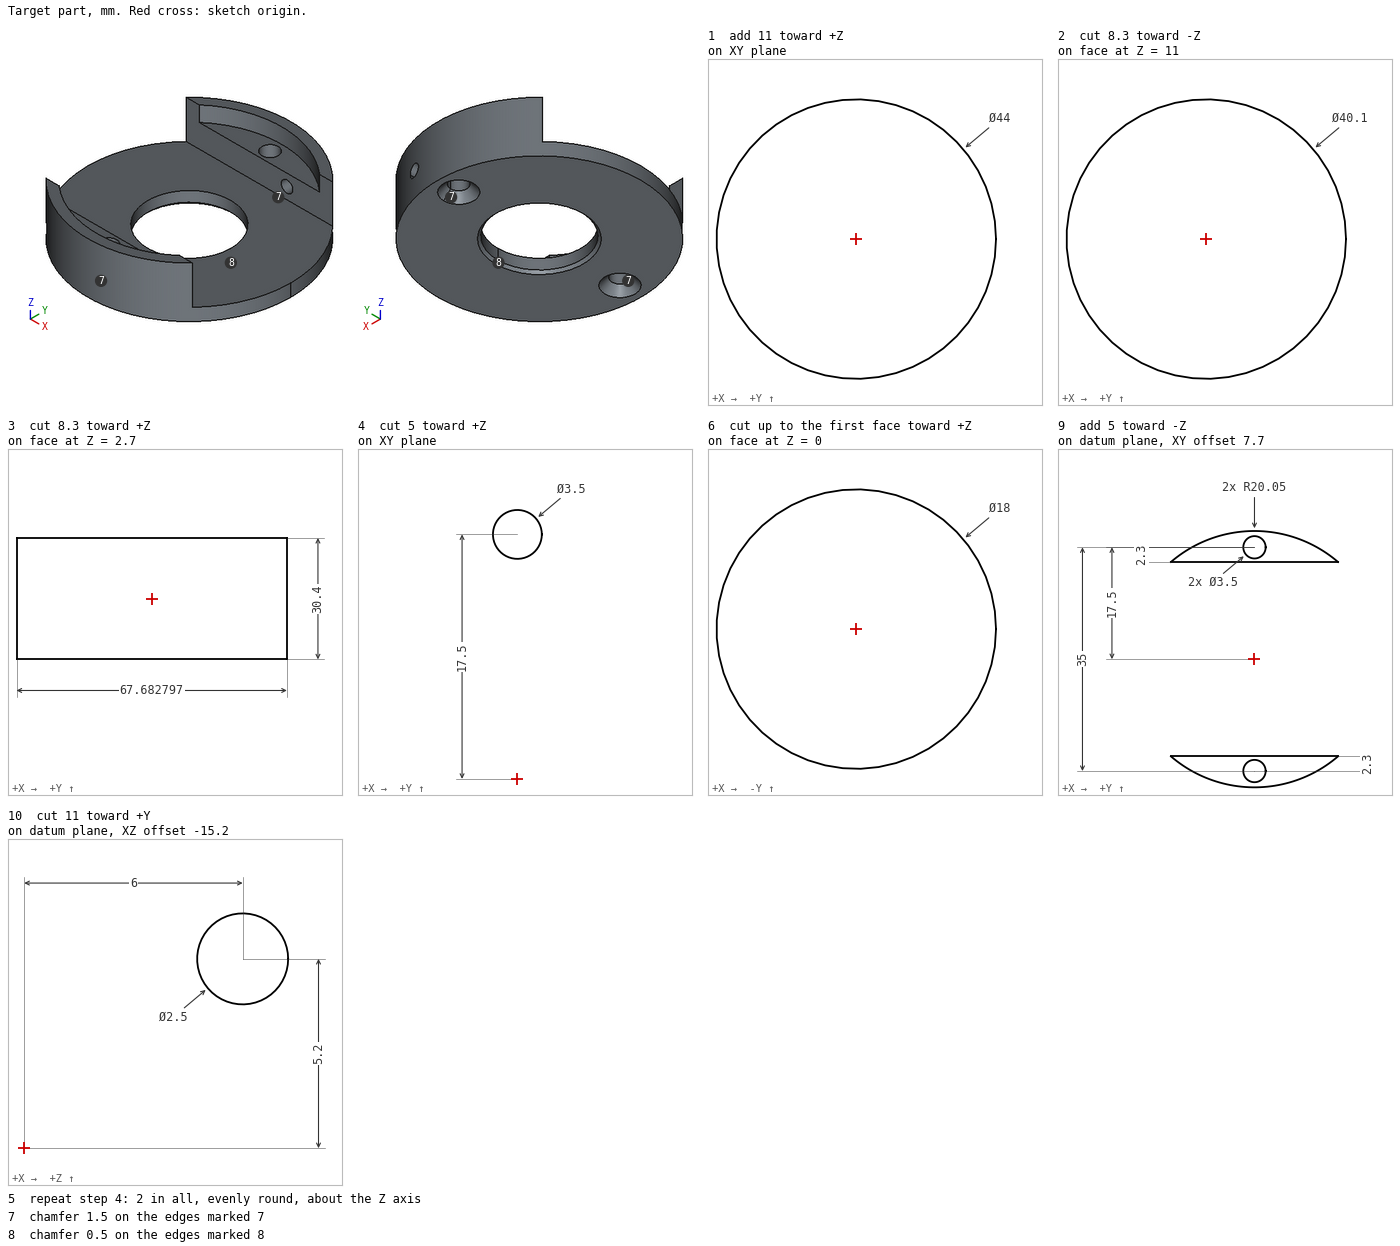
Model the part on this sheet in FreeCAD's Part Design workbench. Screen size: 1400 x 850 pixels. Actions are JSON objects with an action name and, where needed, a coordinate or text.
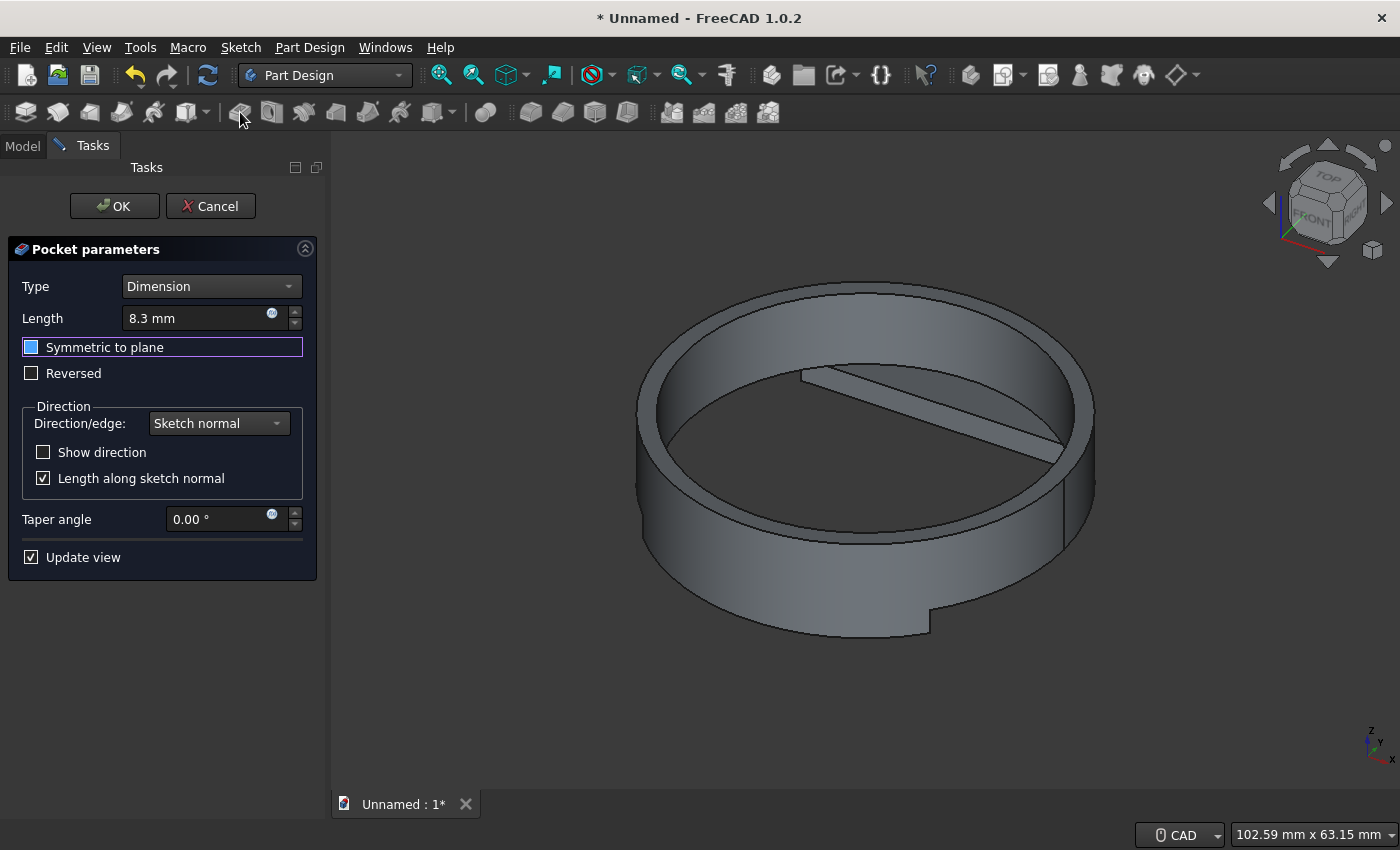
{"action": "left_click", "coordinate": [30, 373]}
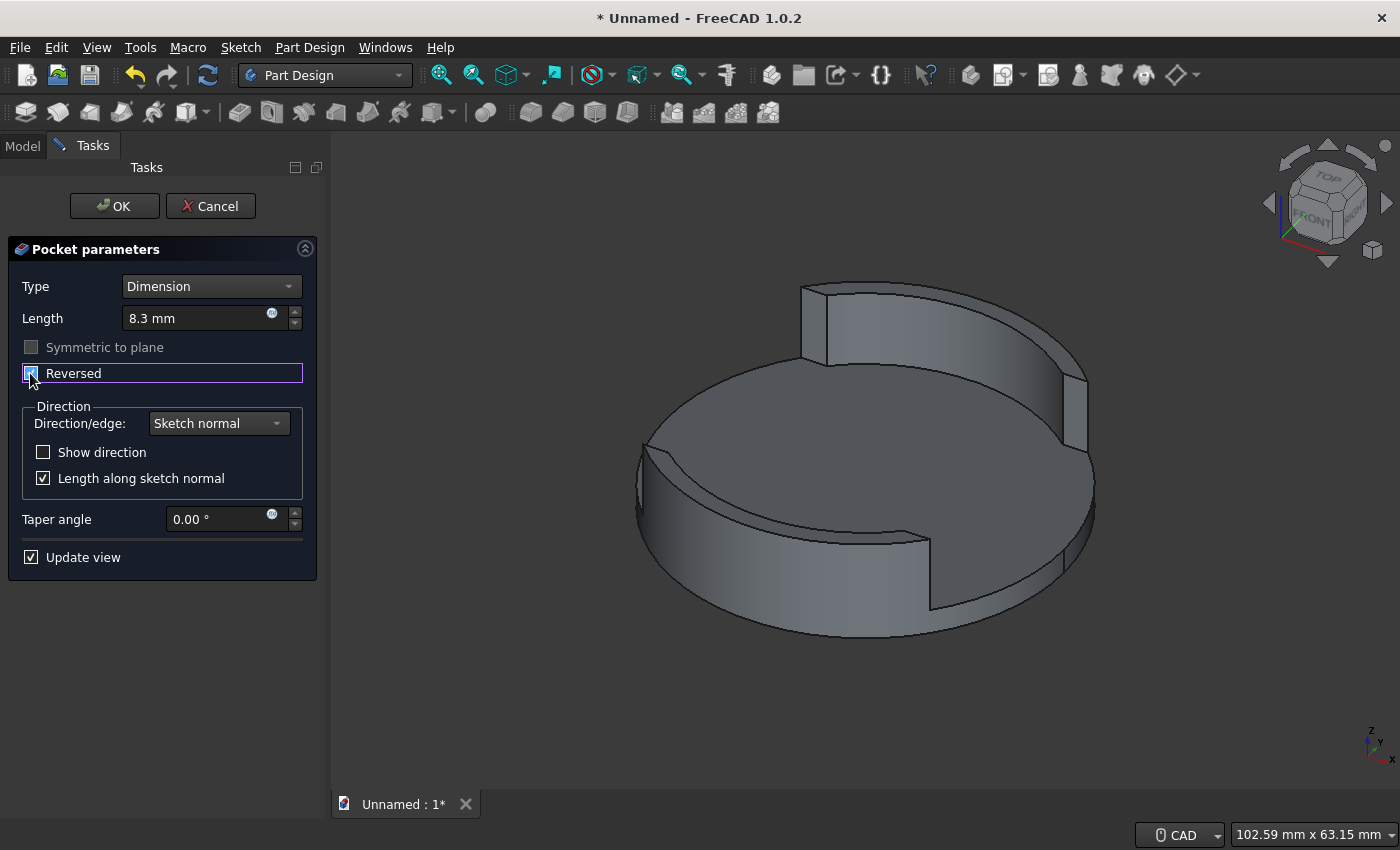
{"action": "left_click", "coordinate": [115, 206]}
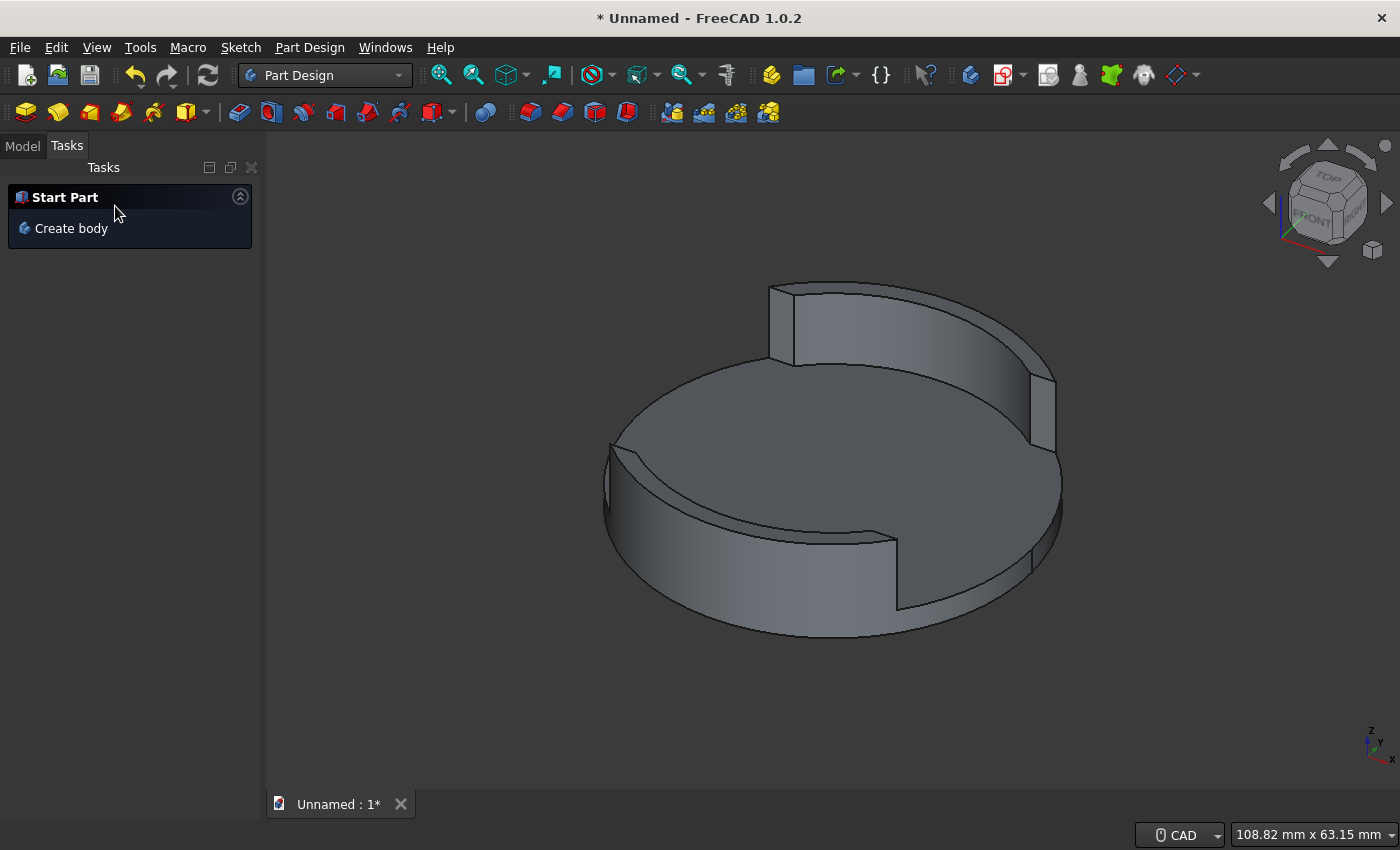
{"action": "left_click", "coordinate": [1004, 76]}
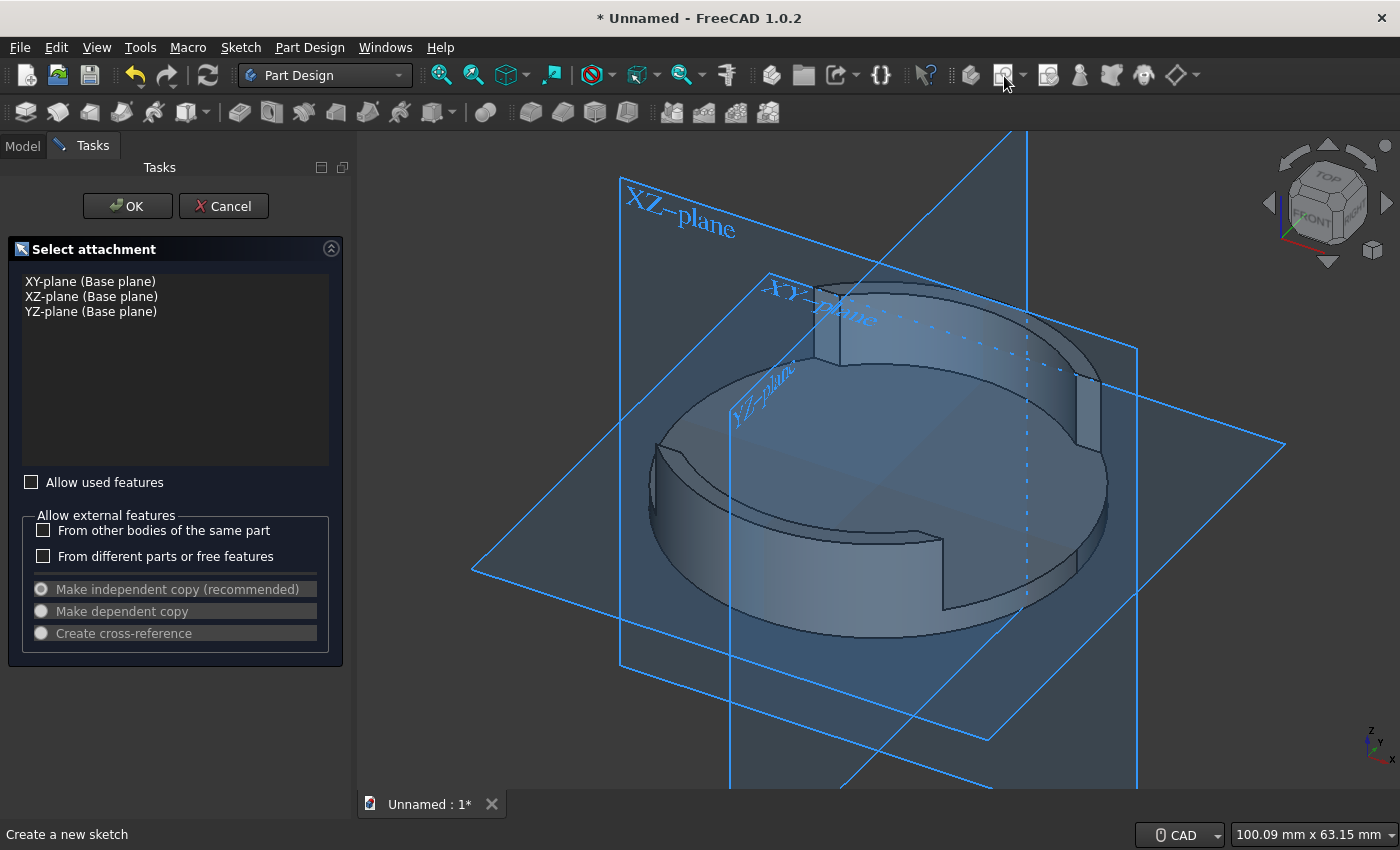
{"action": "left_click", "coordinate": [82, 282]}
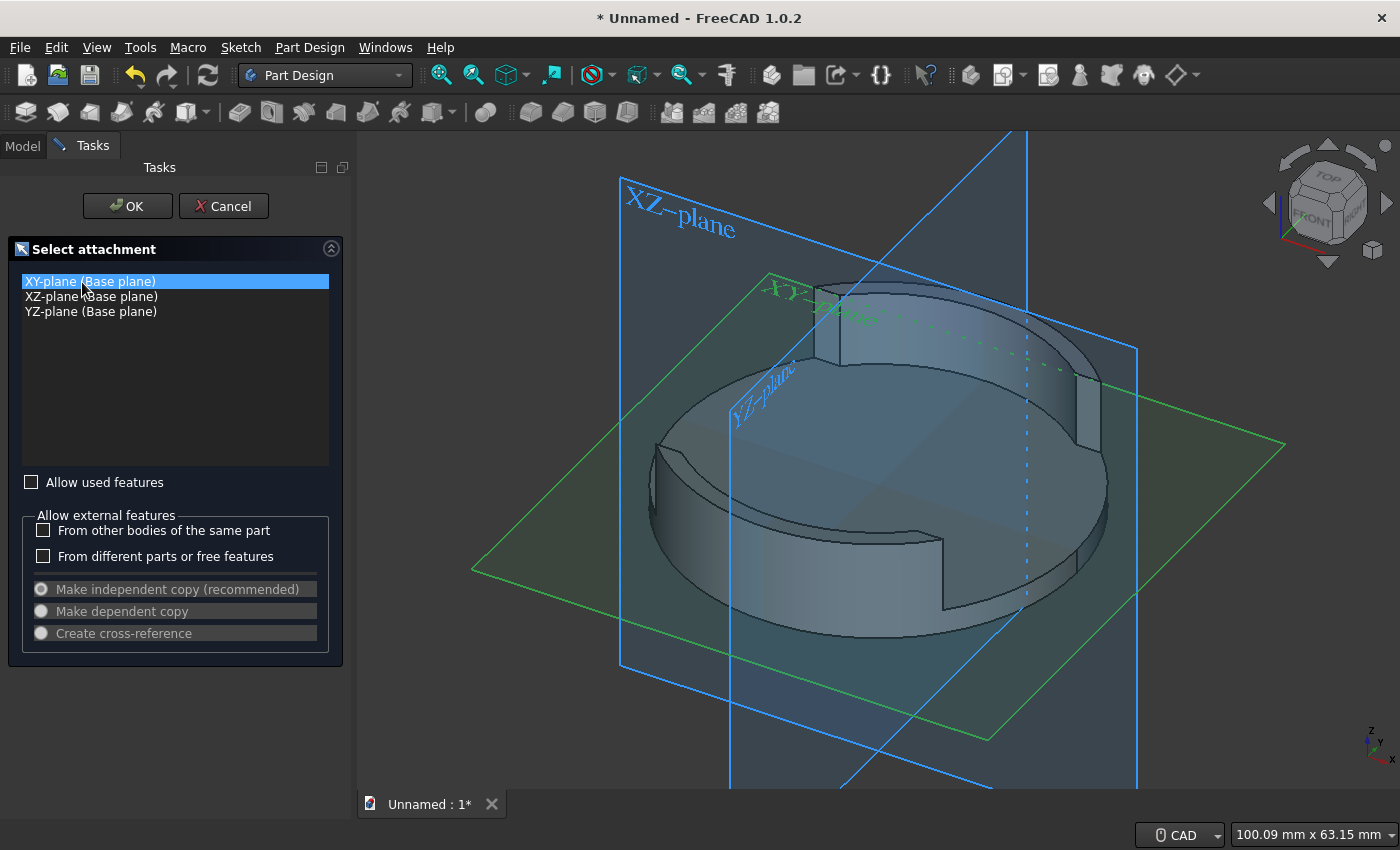
{"action": "left_click", "coordinate": [128, 206]}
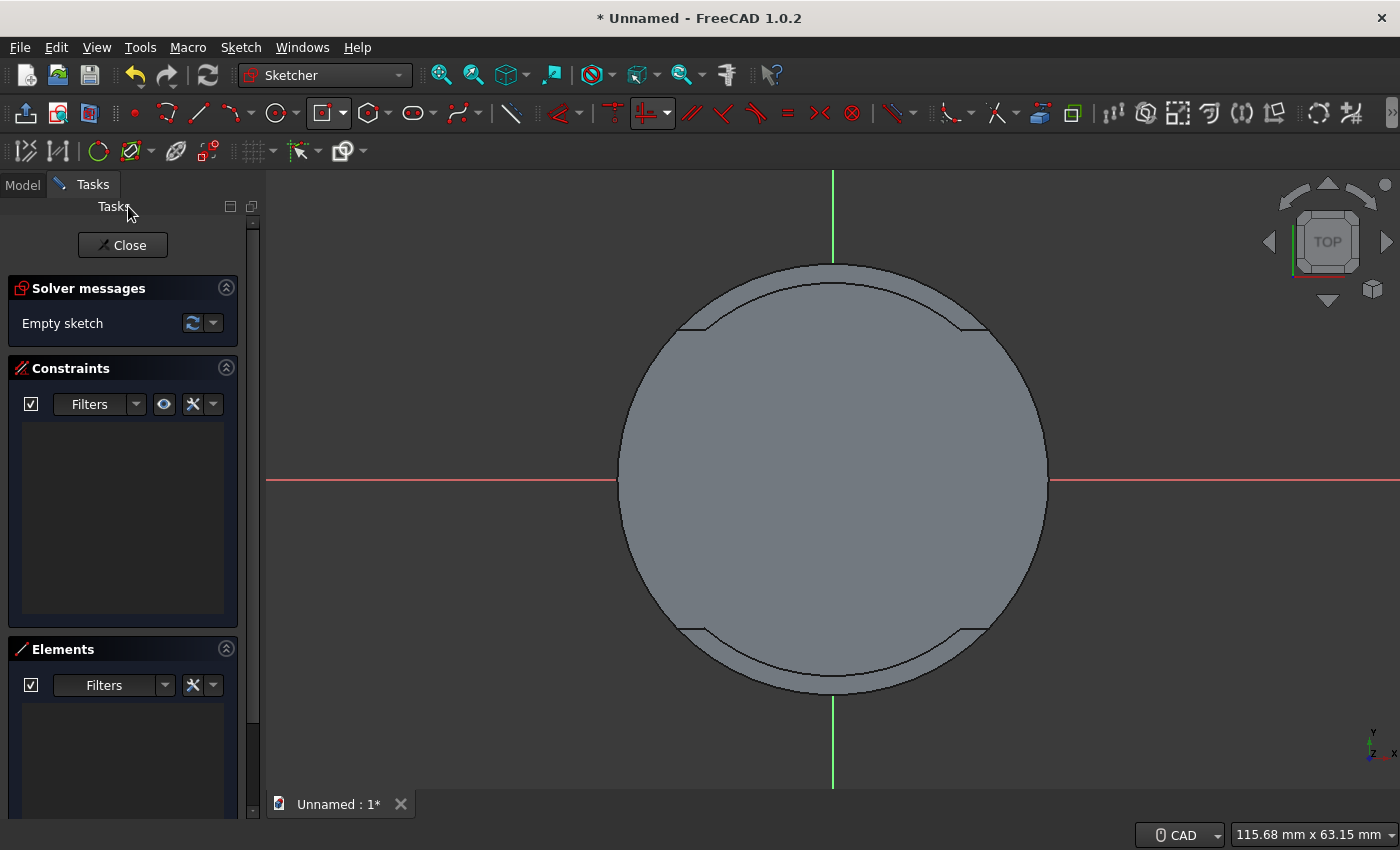
{"action": "key", "text": "q s"}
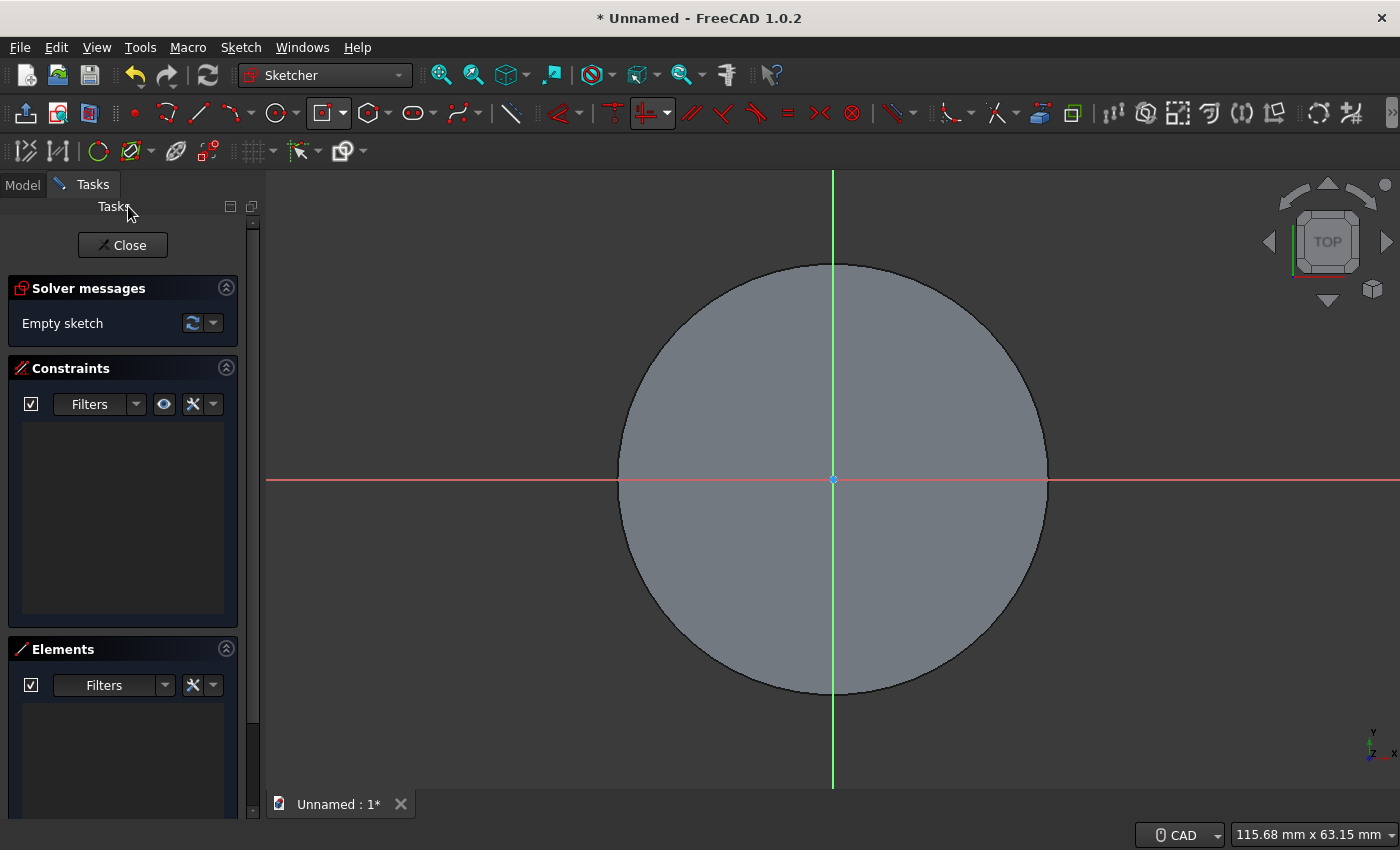
{"action": "scroll", "coordinate": [840, 291], "scroll_direction": "up", "scroll_amount": 12}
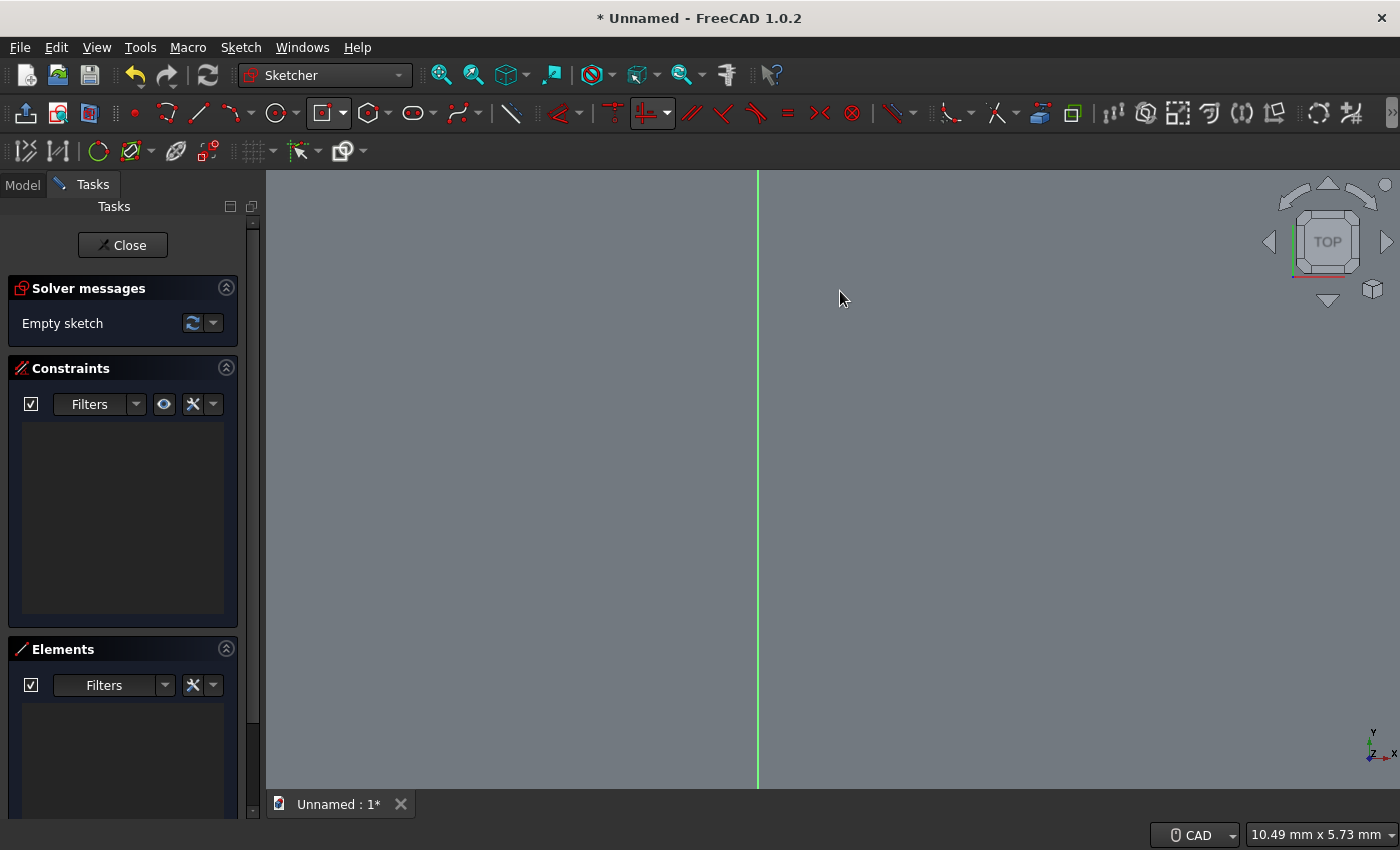
{"action": "left_click", "coordinate": [276, 114]}